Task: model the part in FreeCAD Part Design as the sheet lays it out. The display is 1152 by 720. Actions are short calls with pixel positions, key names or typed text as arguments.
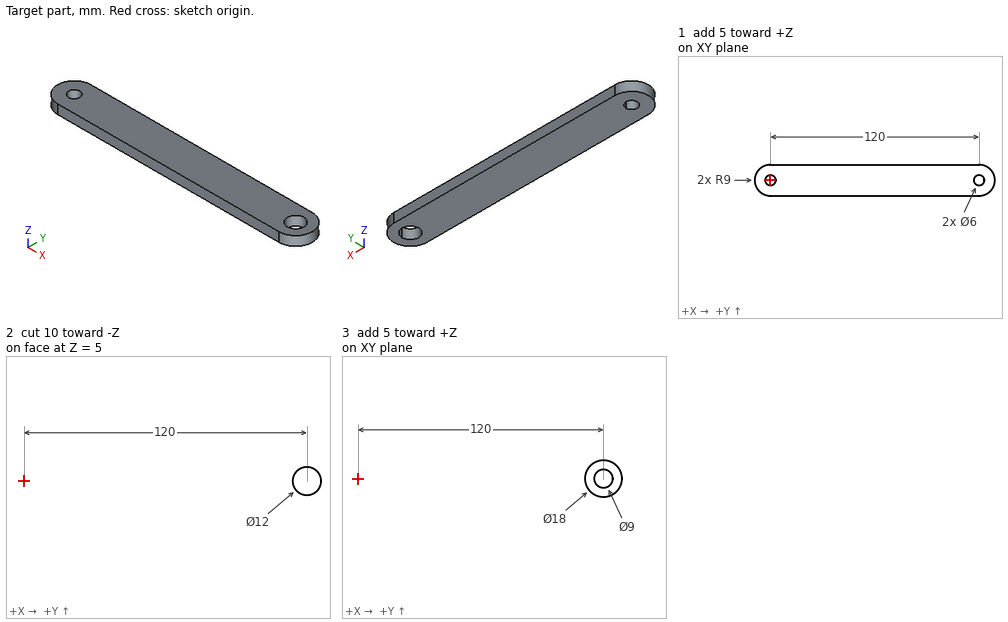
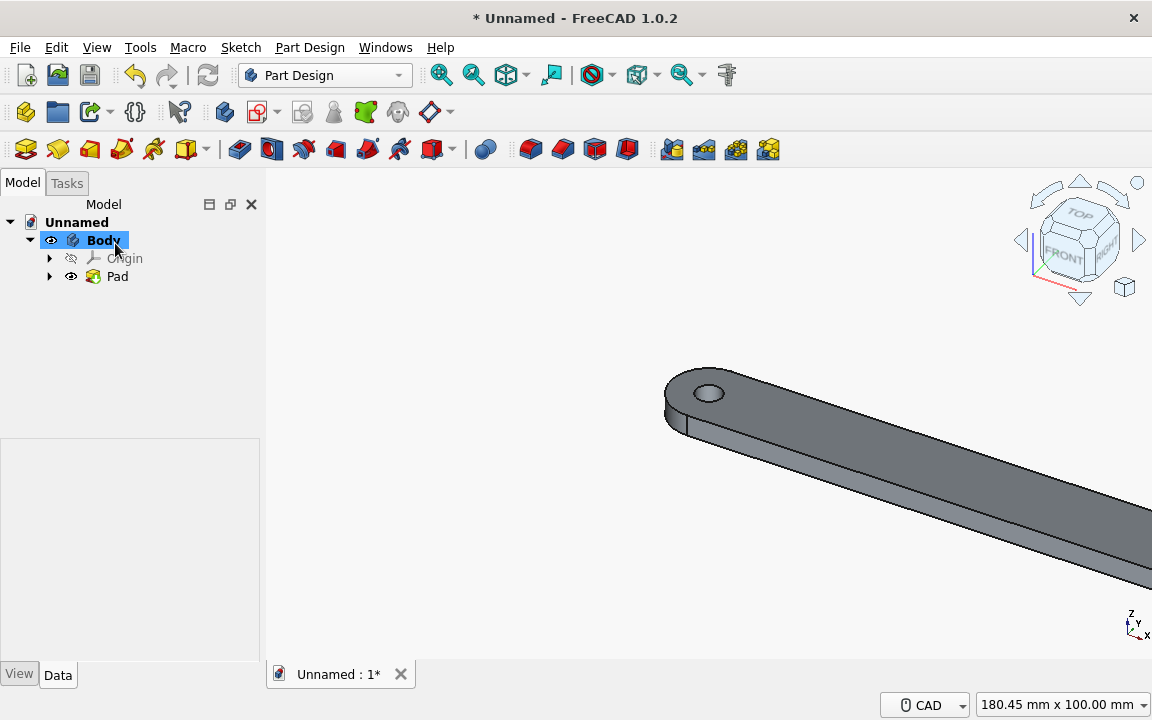
click(442, 76)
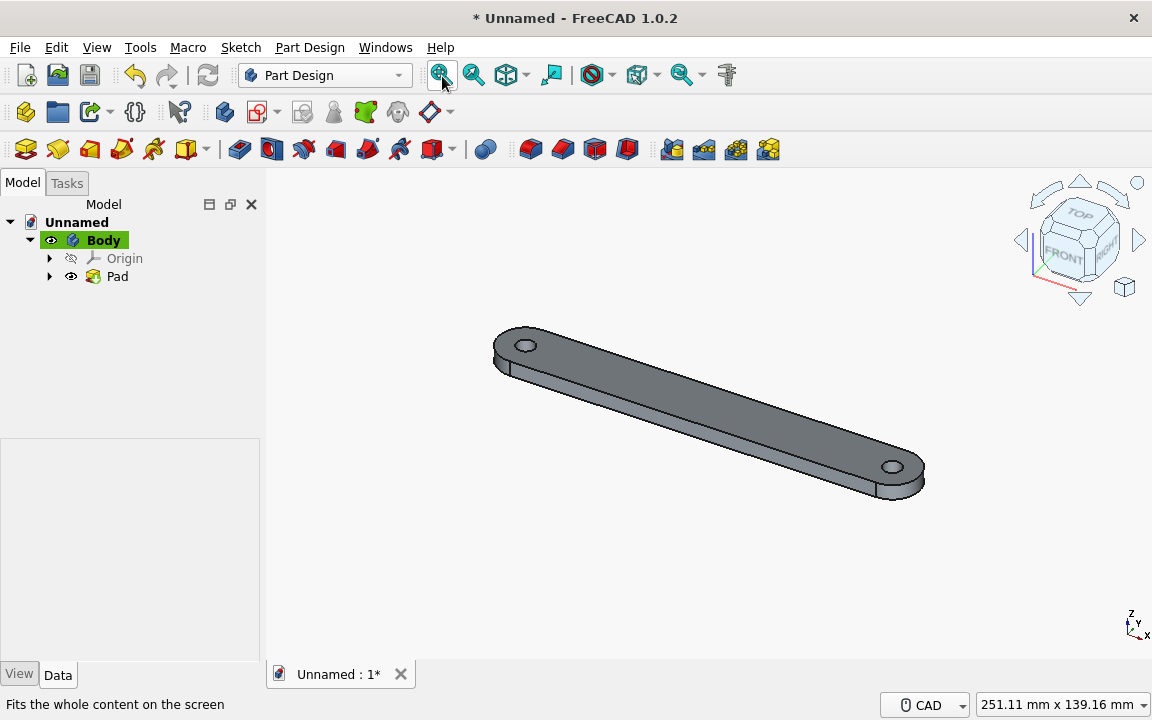
click(829, 445)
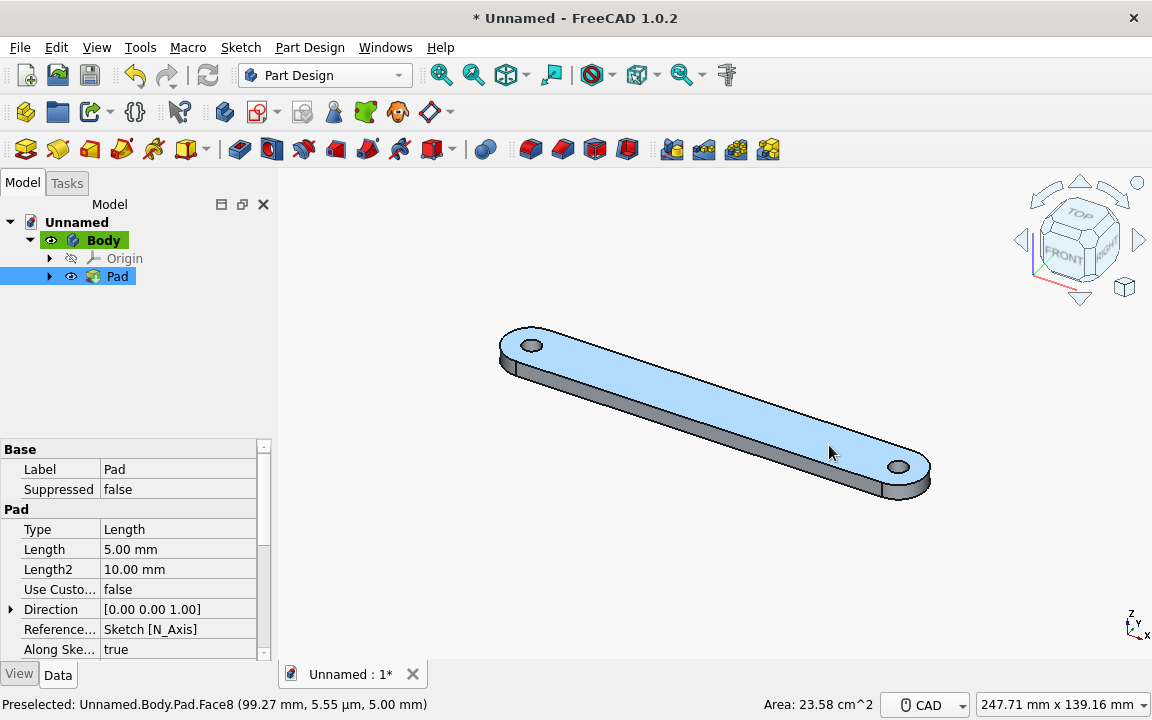
click(258, 112)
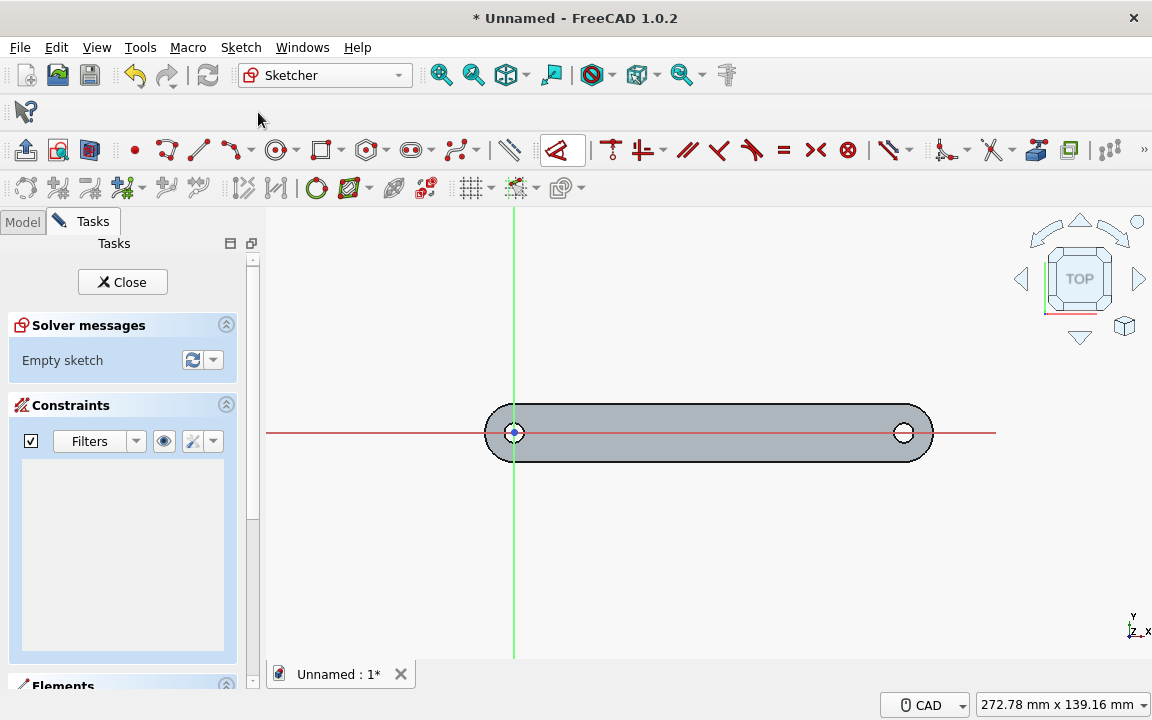
scroll(945, 433, up, 10)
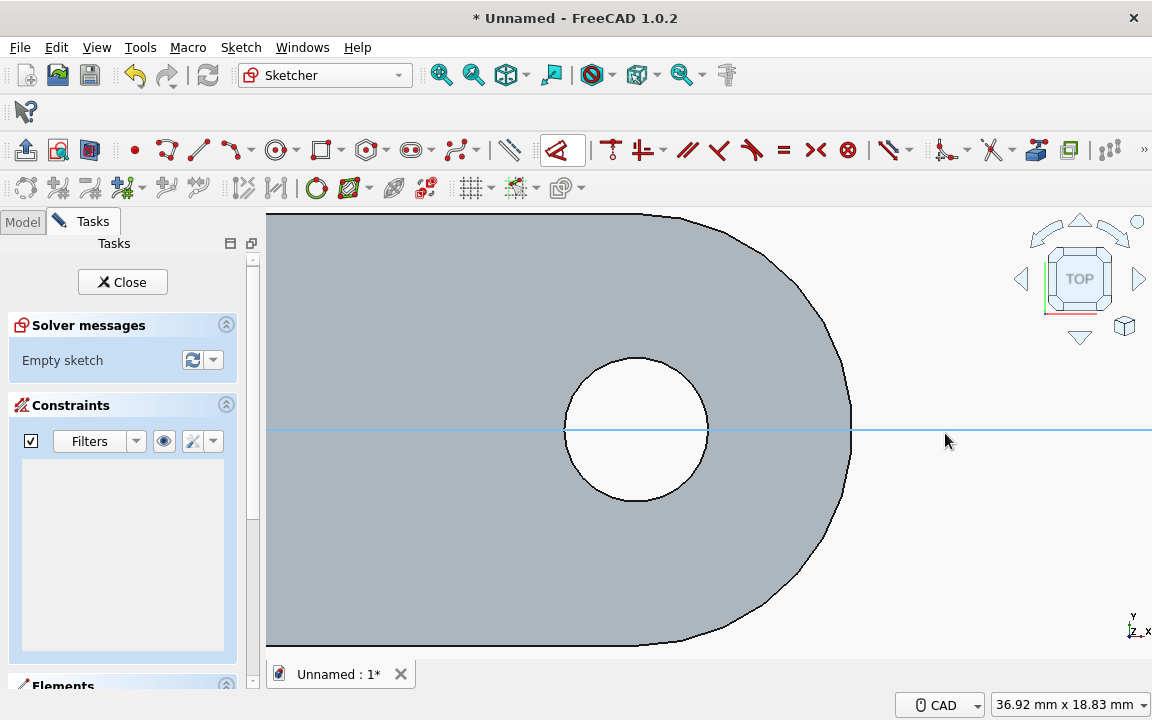
click(276, 150)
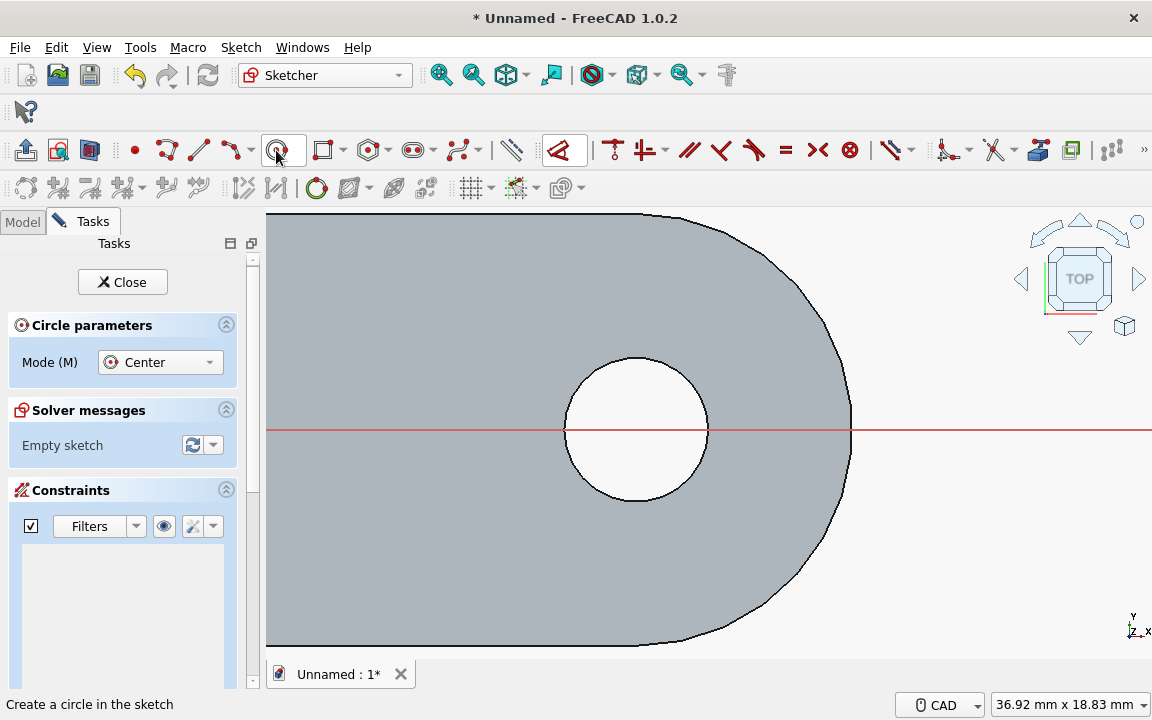
click(636, 430)
move(738, 328)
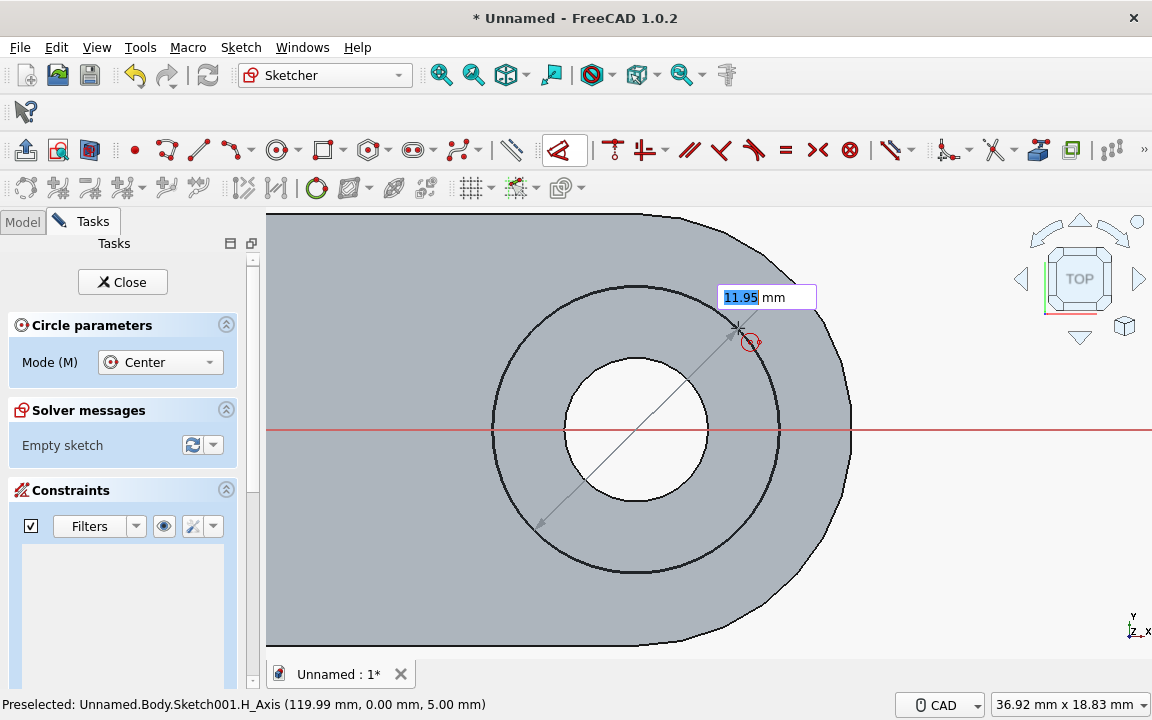
text(12)
key(Return)
key(Escape)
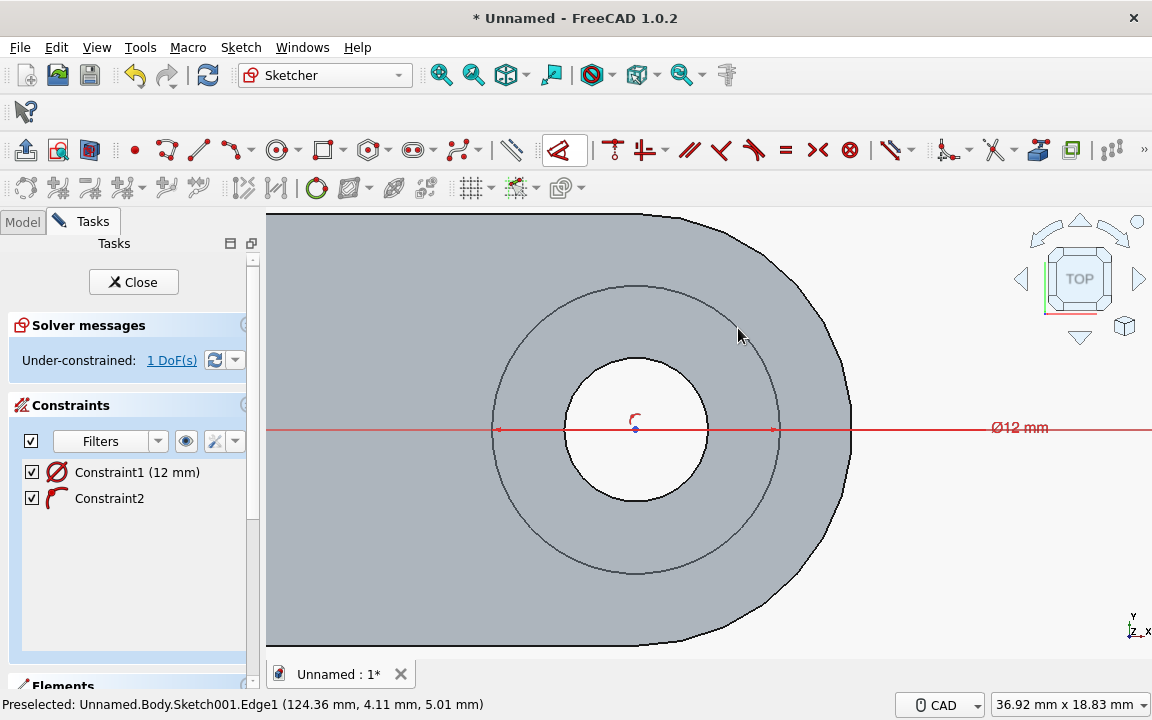
click(636, 430)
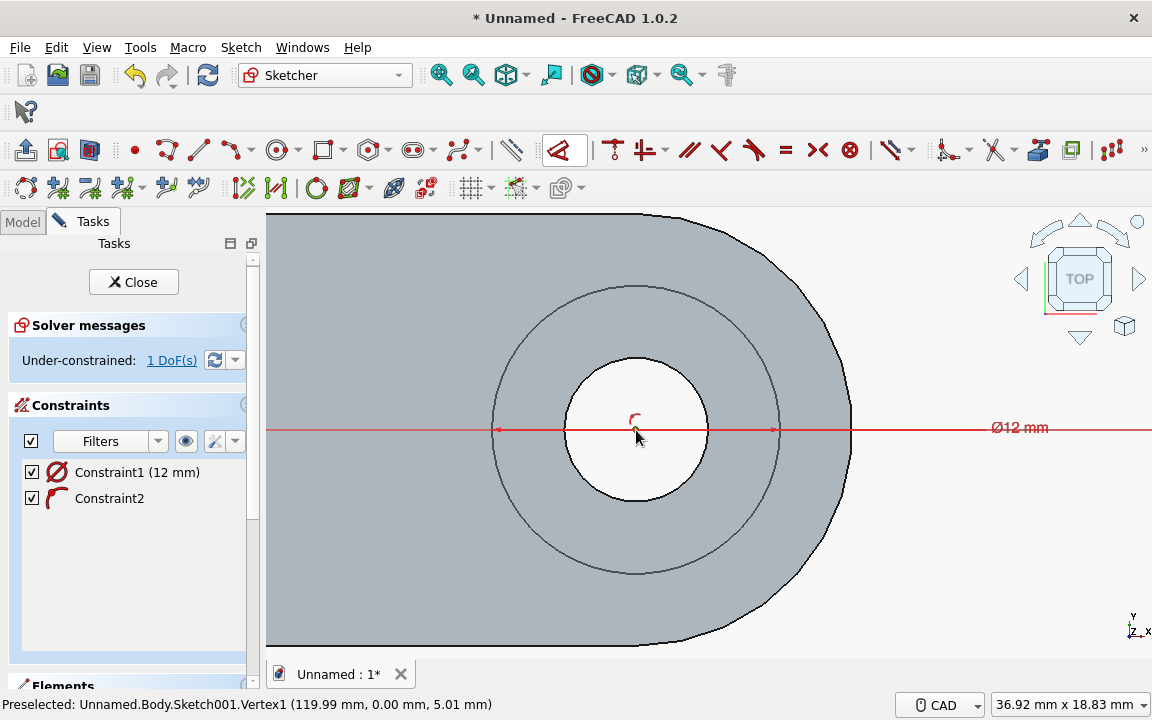
key(l)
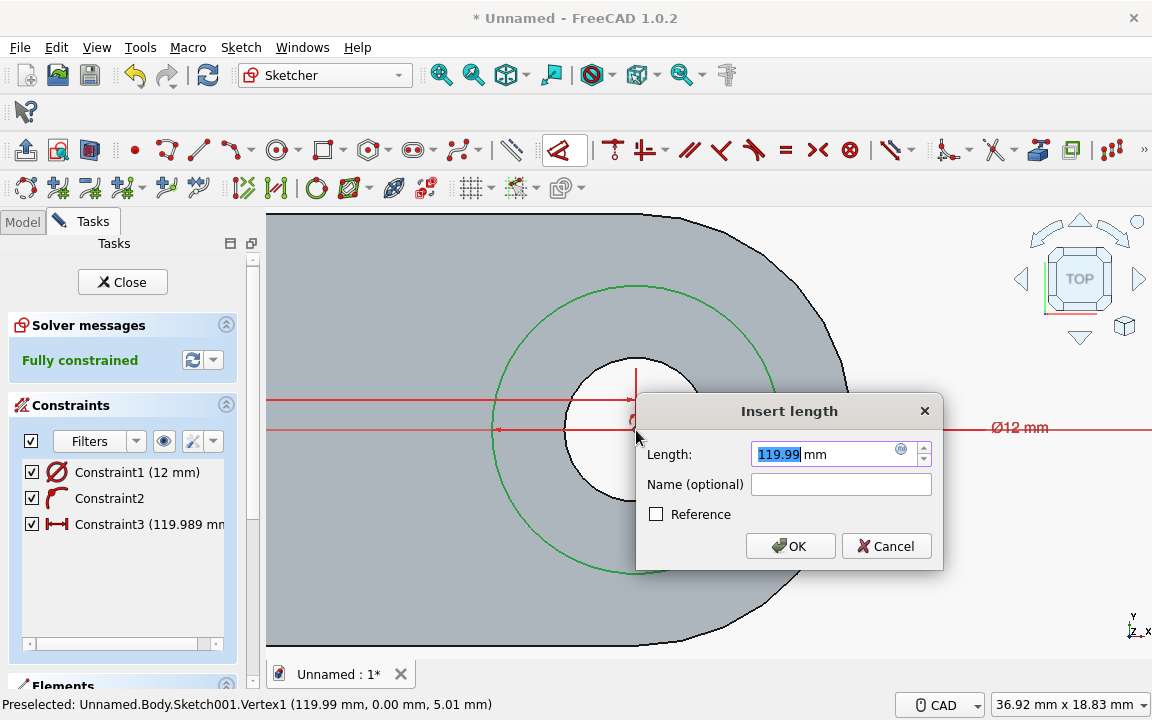
text(120)
key(Return)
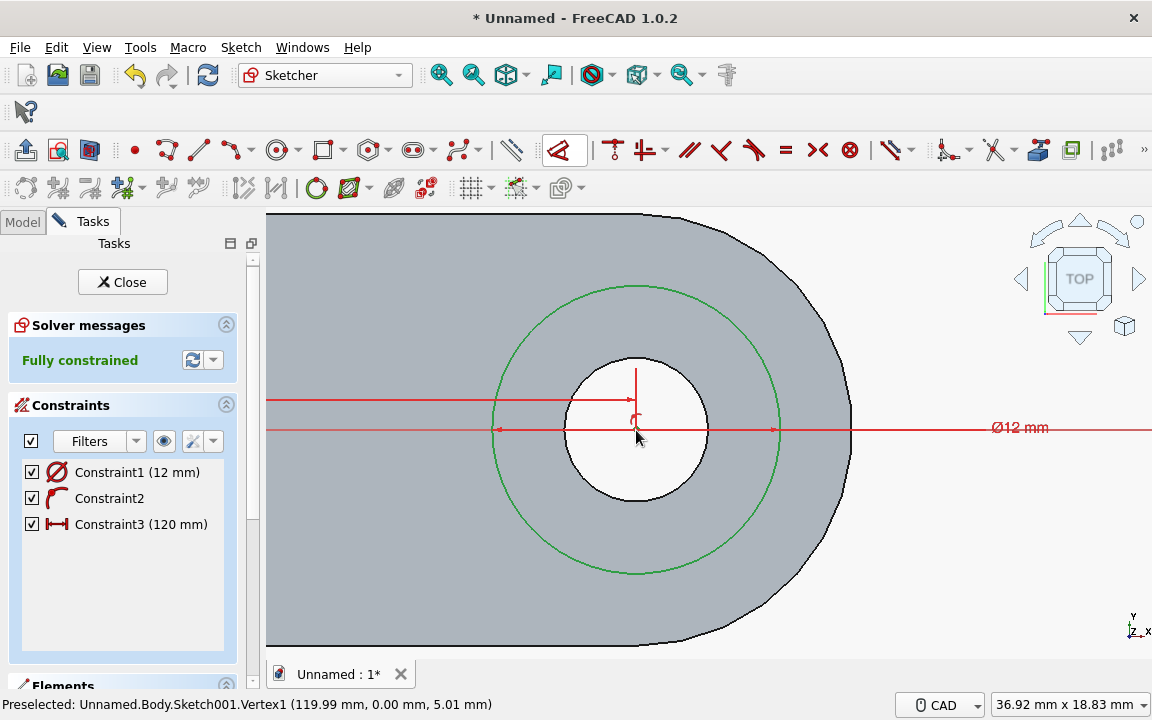
click(123, 282)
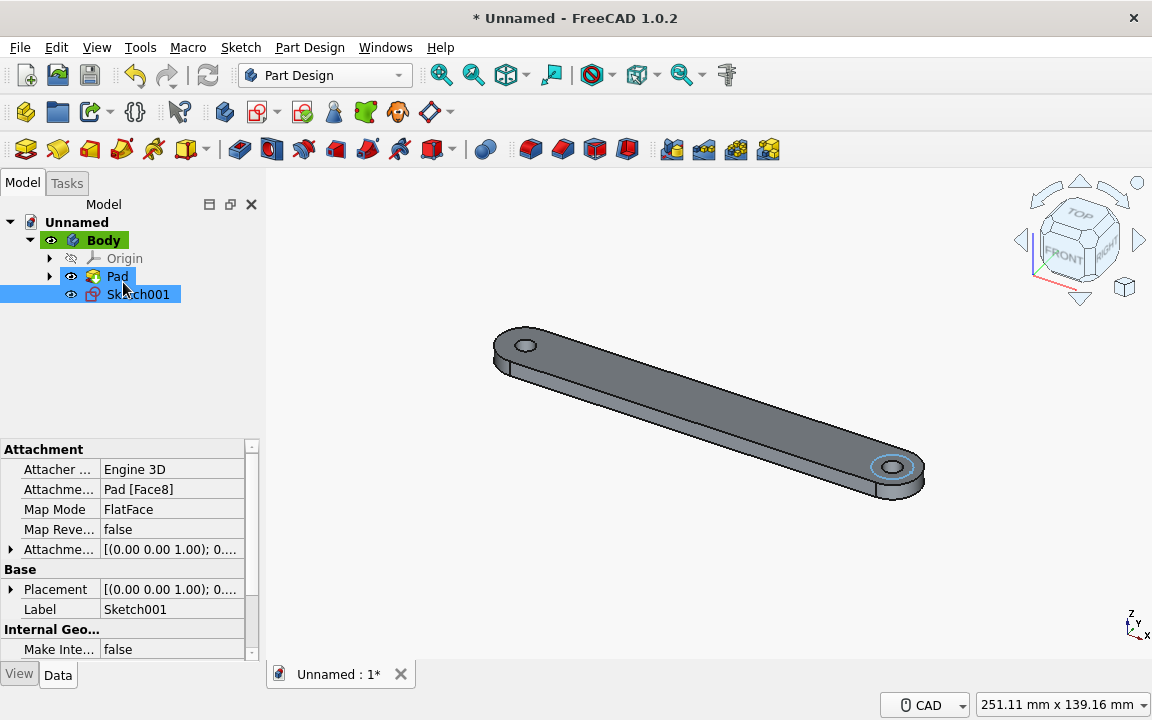
click(240, 150)